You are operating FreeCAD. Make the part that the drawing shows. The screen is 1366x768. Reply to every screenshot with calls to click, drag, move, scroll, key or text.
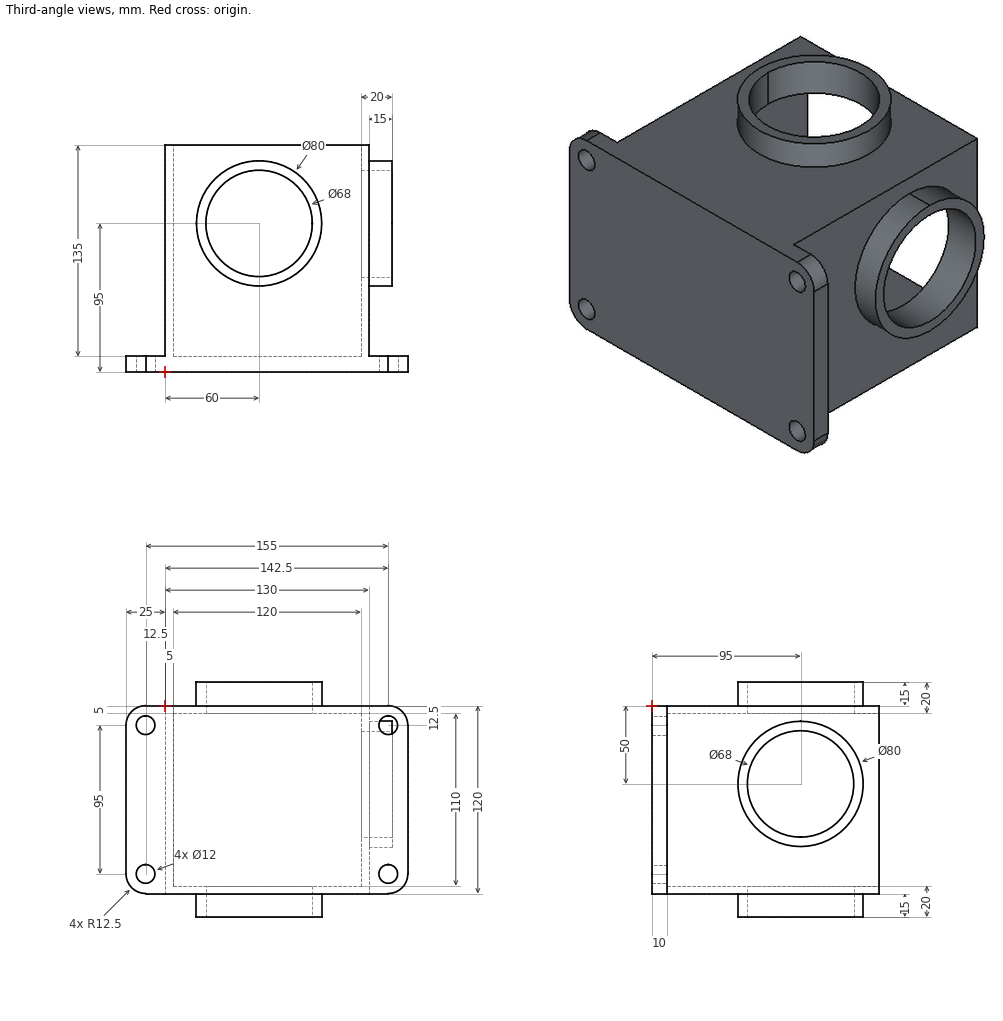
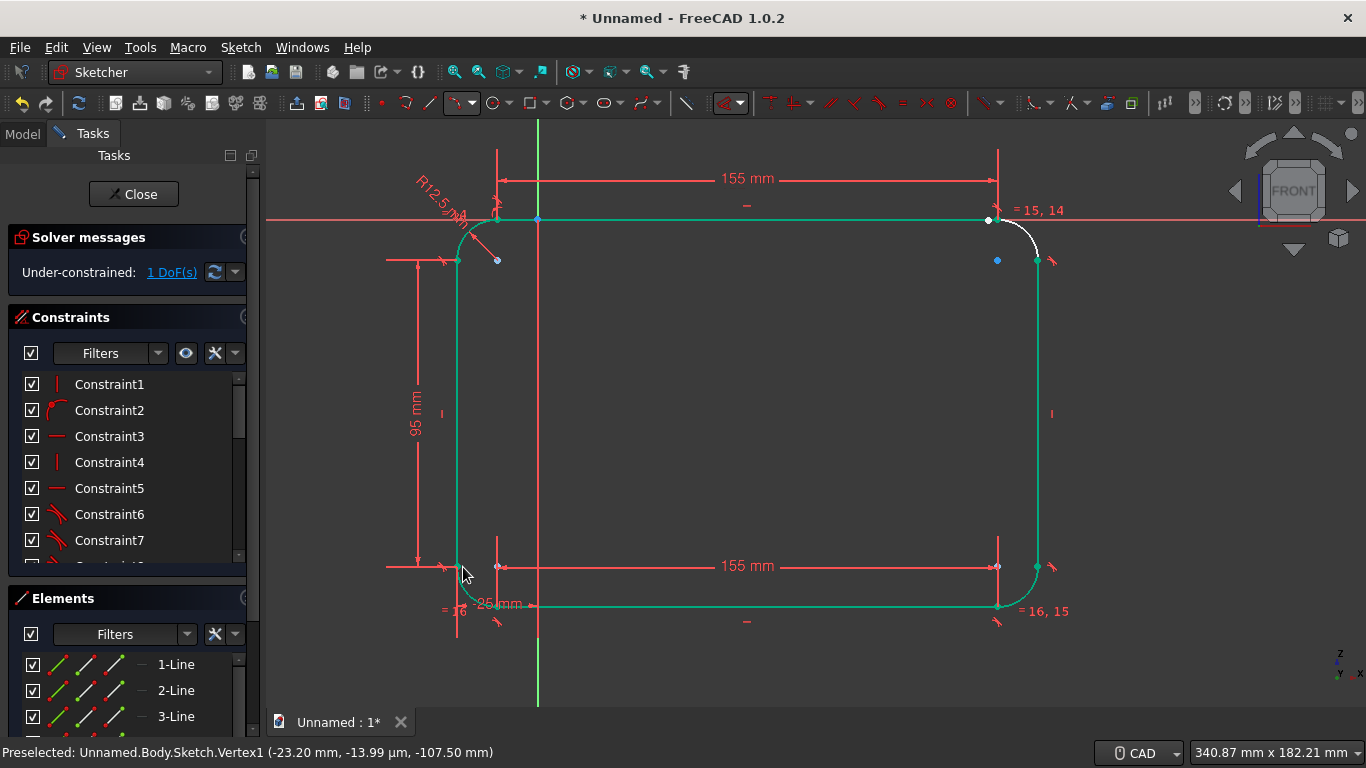
click(989, 221)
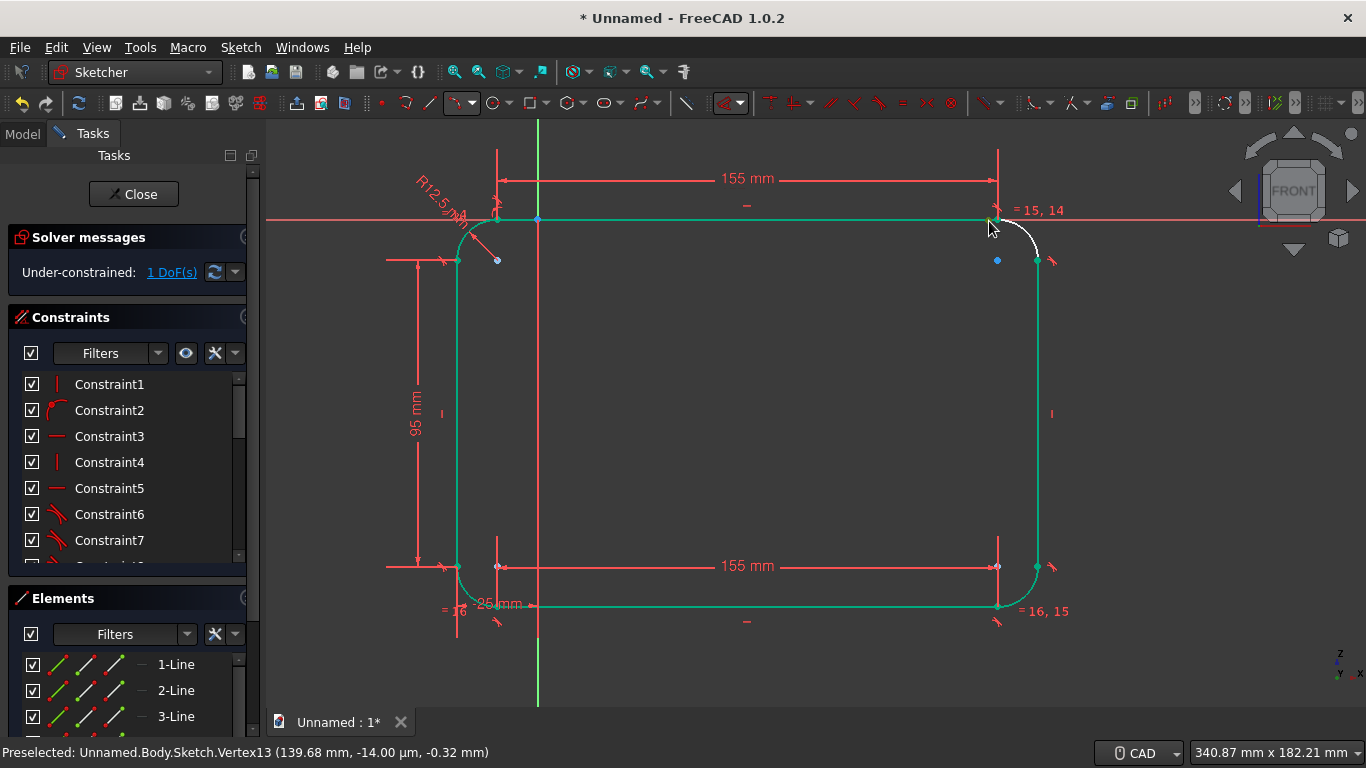
click(742, 104)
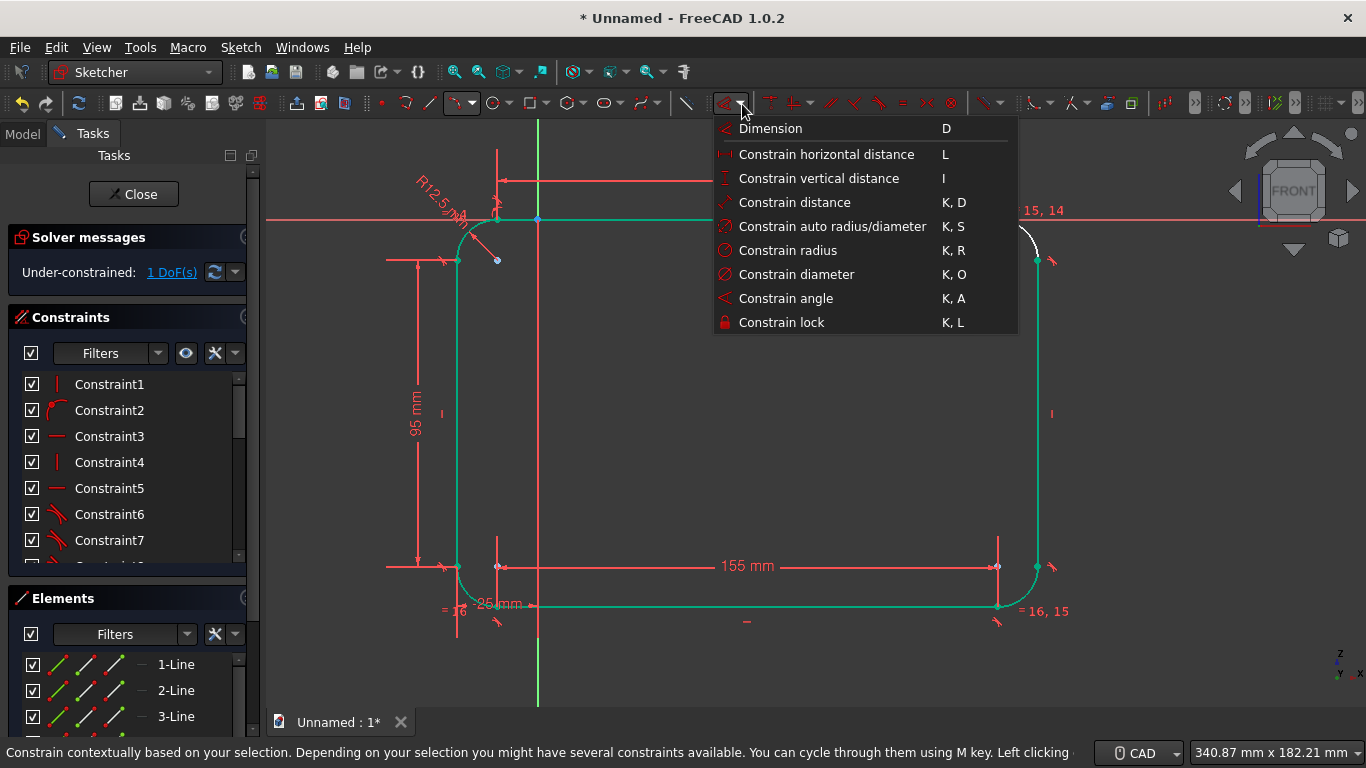
click(866, 154)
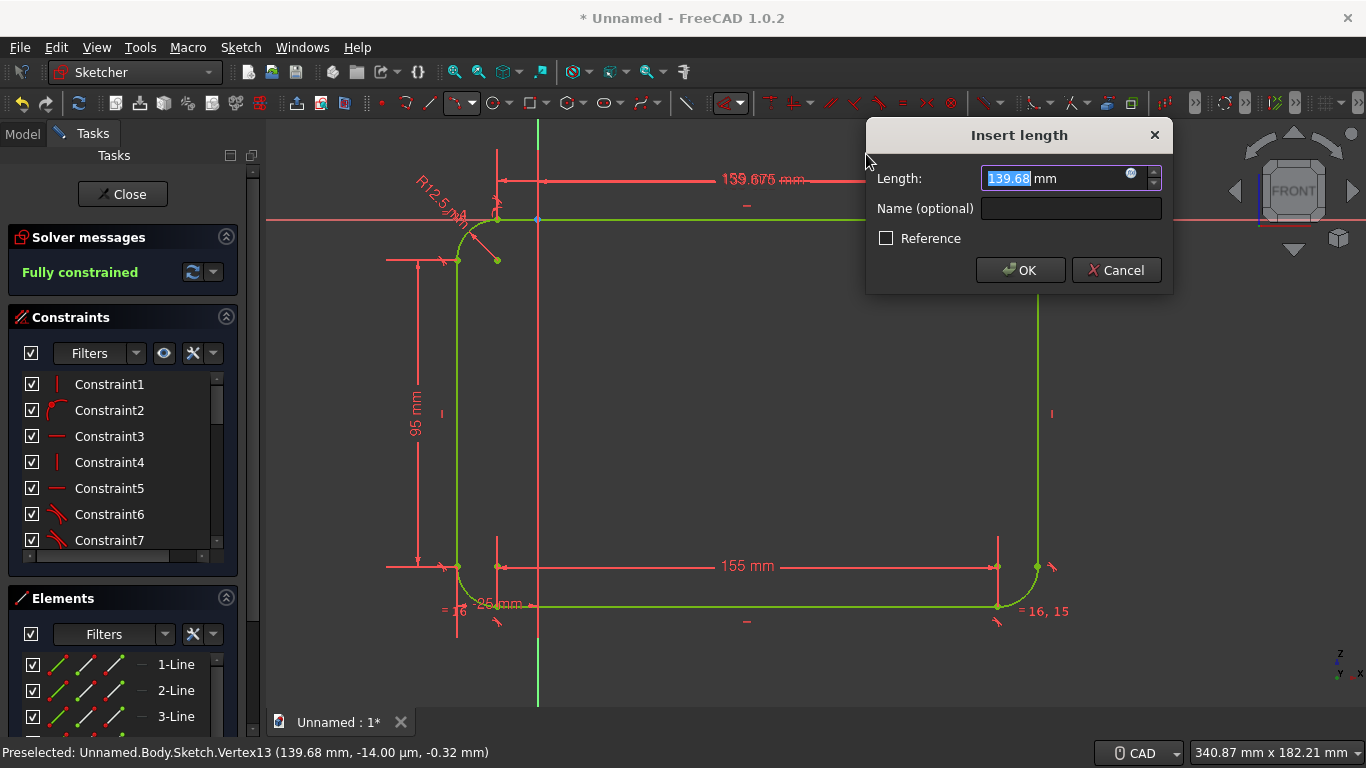
text(142.5)
key(Return)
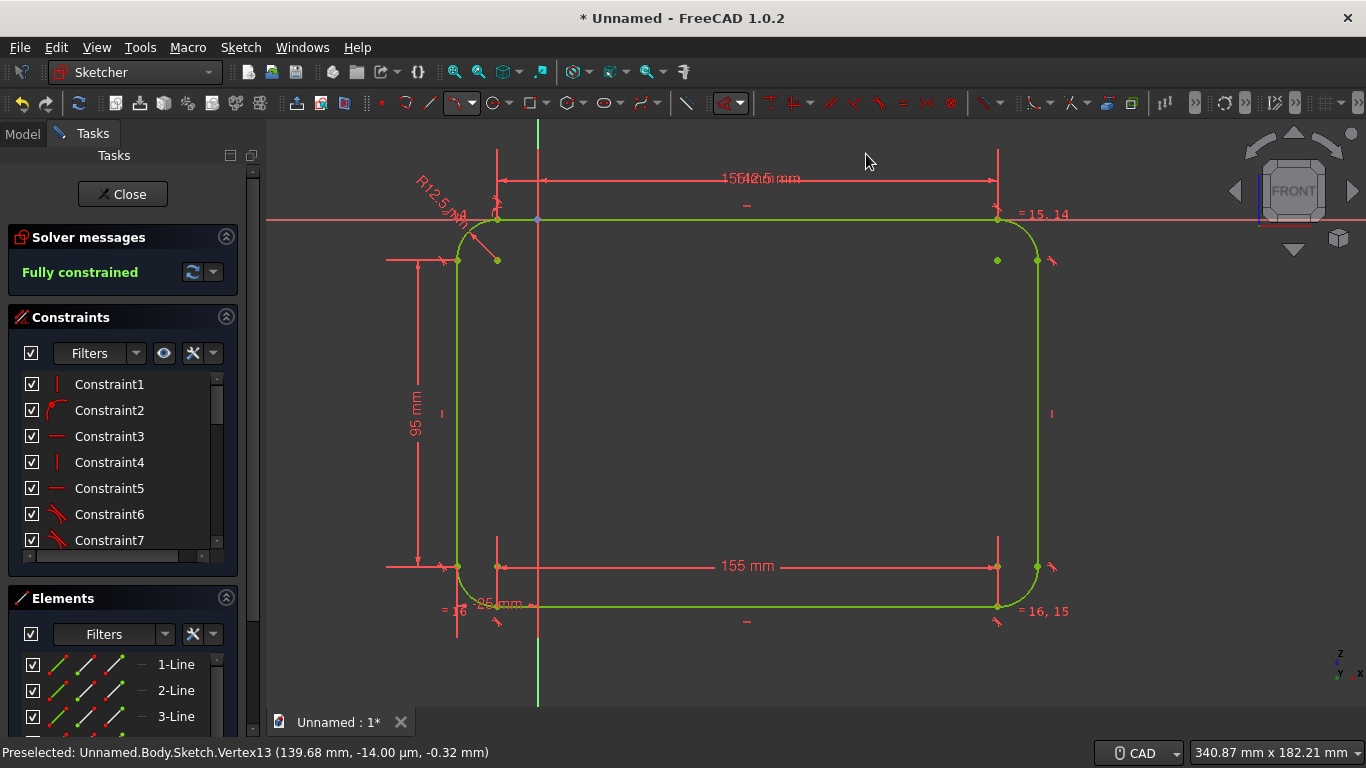
click(123, 194)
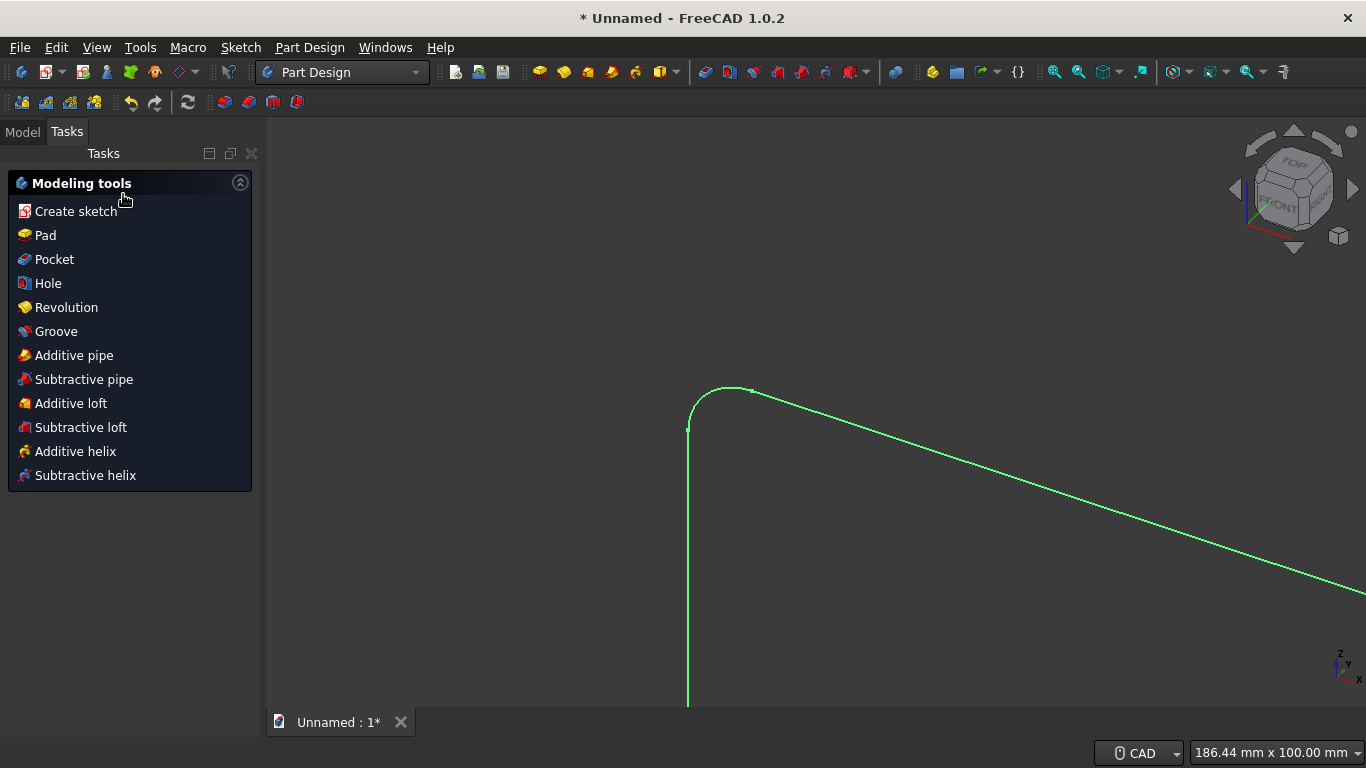
click(540, 72)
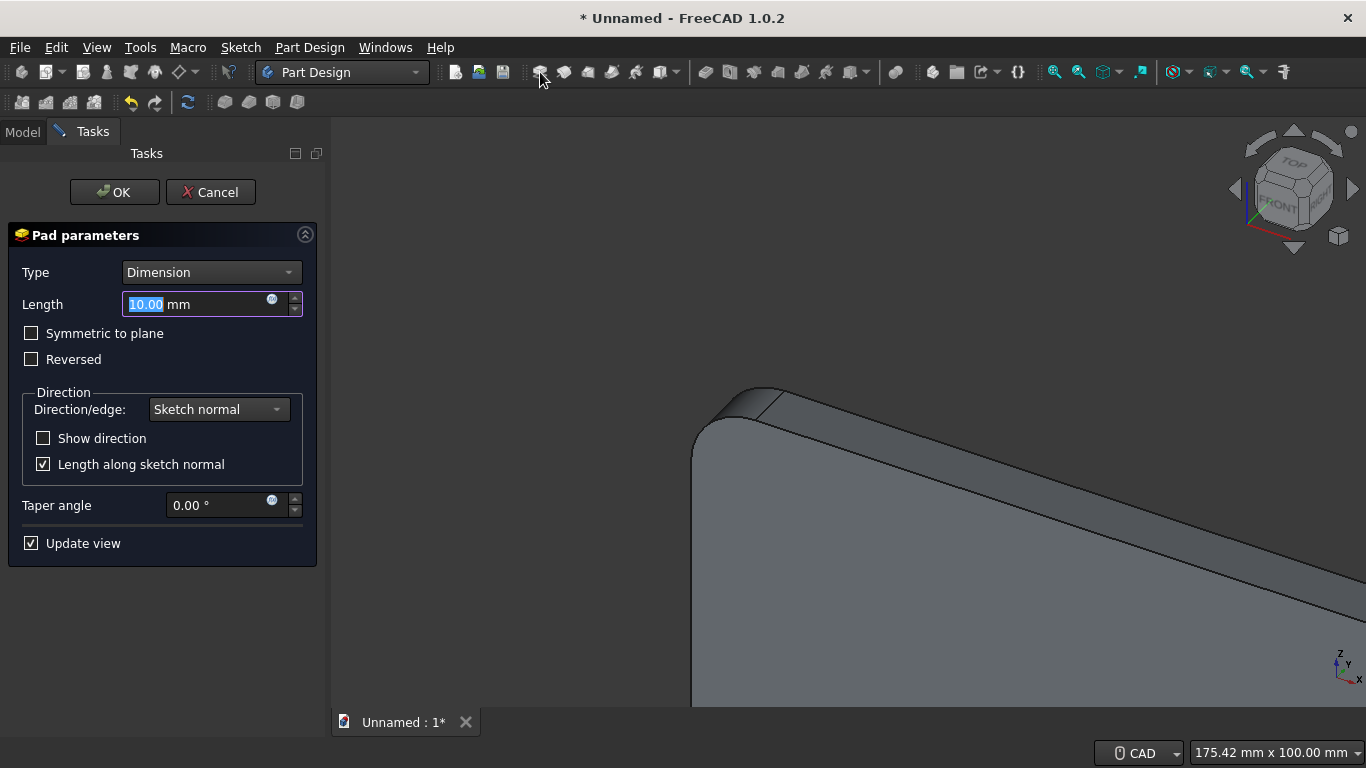
text(10)
key(Tab)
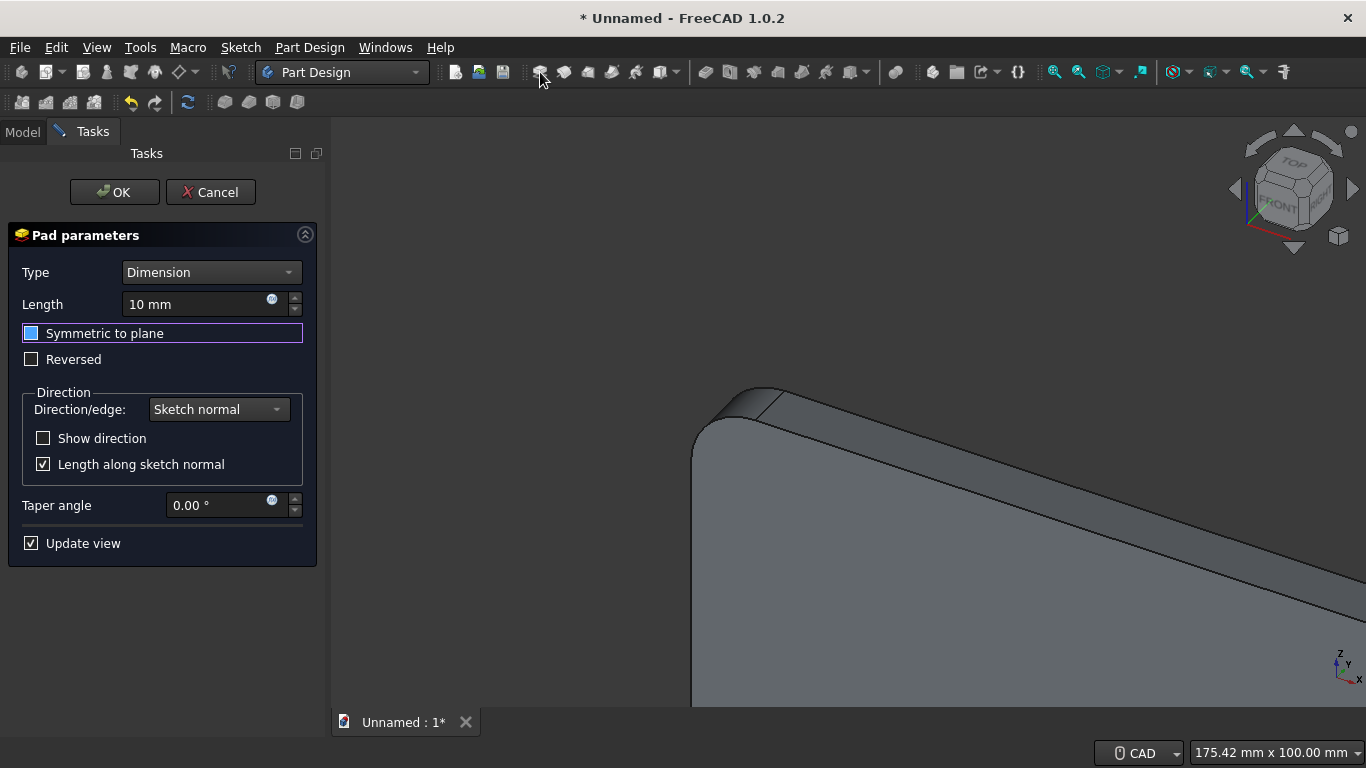
click(30, 359)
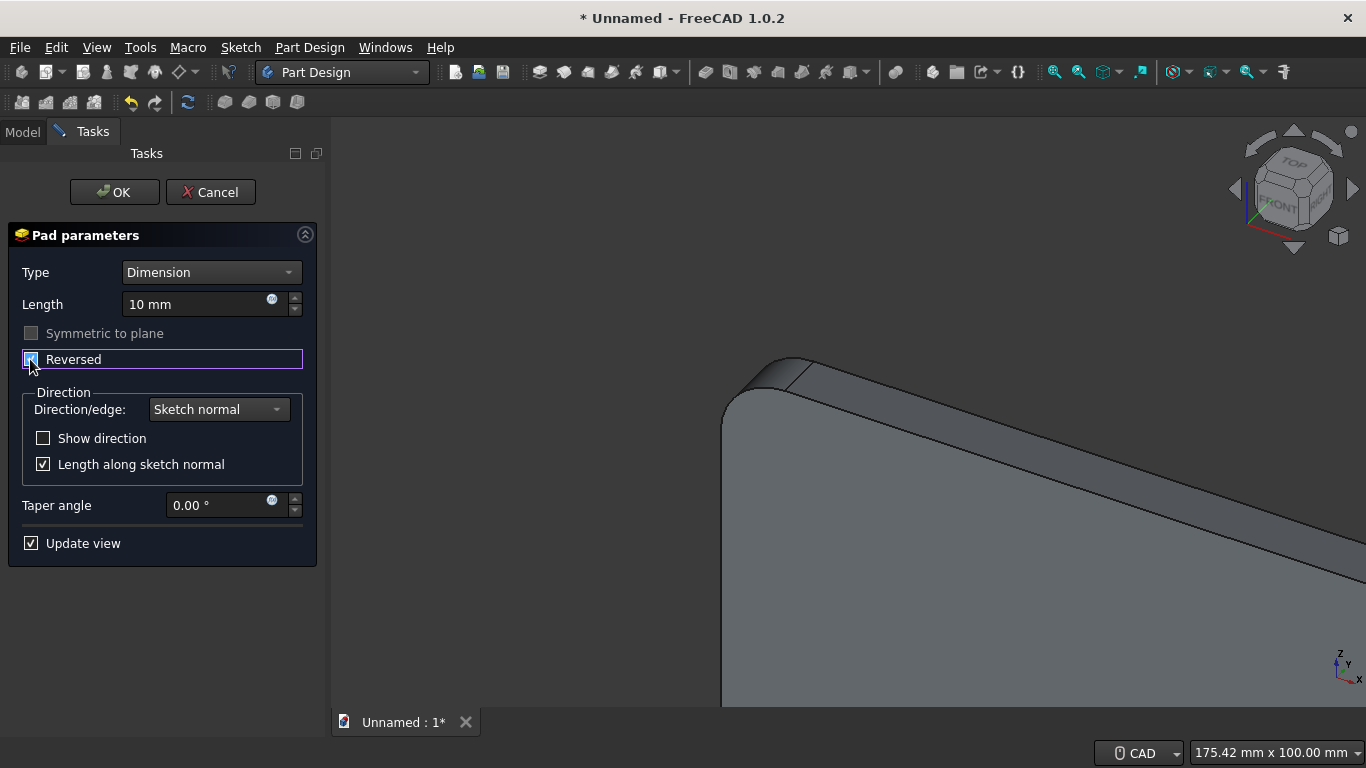
click(115, 192)